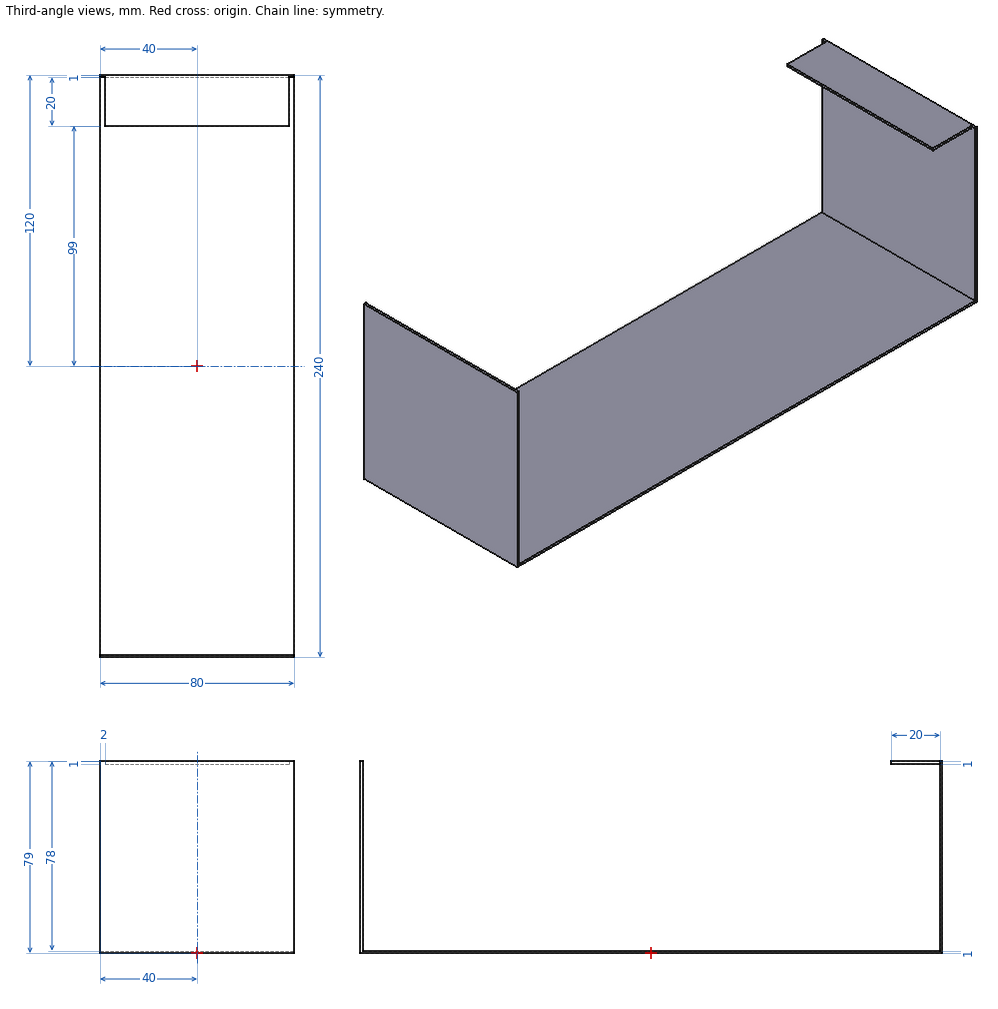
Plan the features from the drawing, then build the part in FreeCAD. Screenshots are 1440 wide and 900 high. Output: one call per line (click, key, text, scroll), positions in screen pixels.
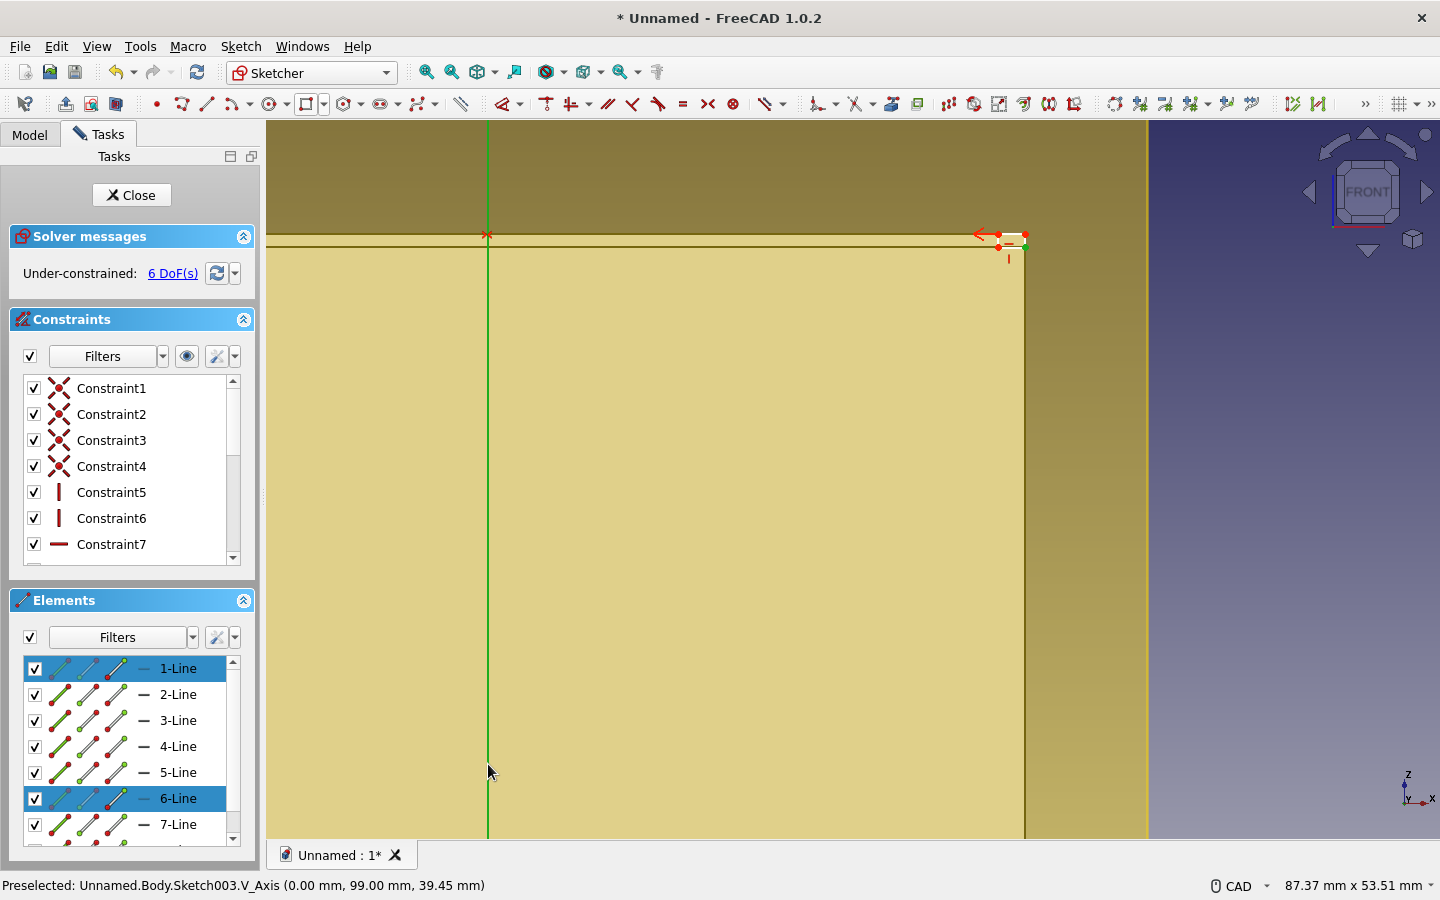
click(708, 104)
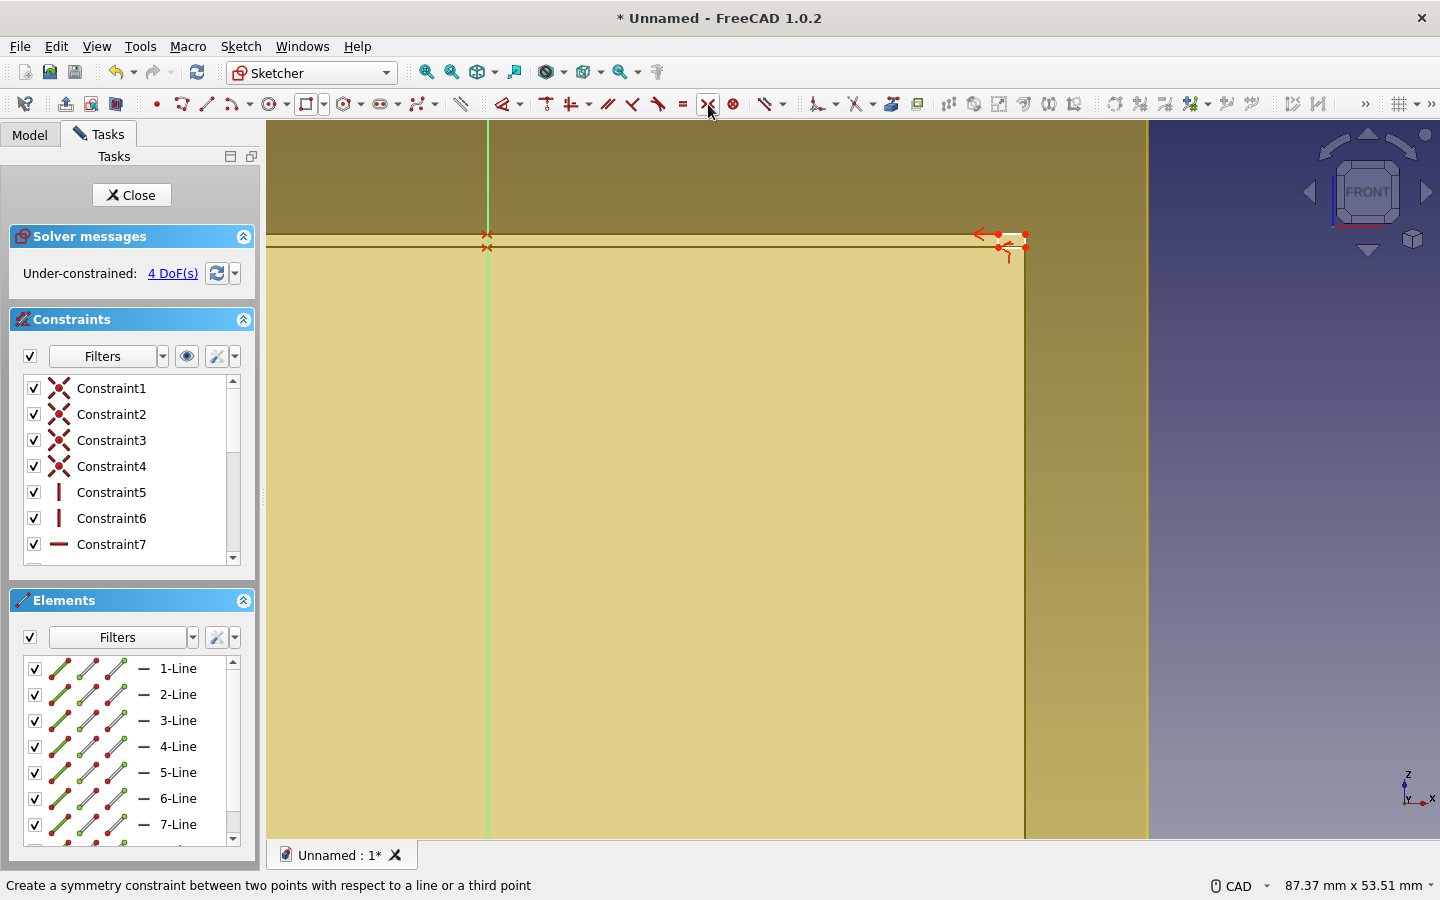
click(502, 104)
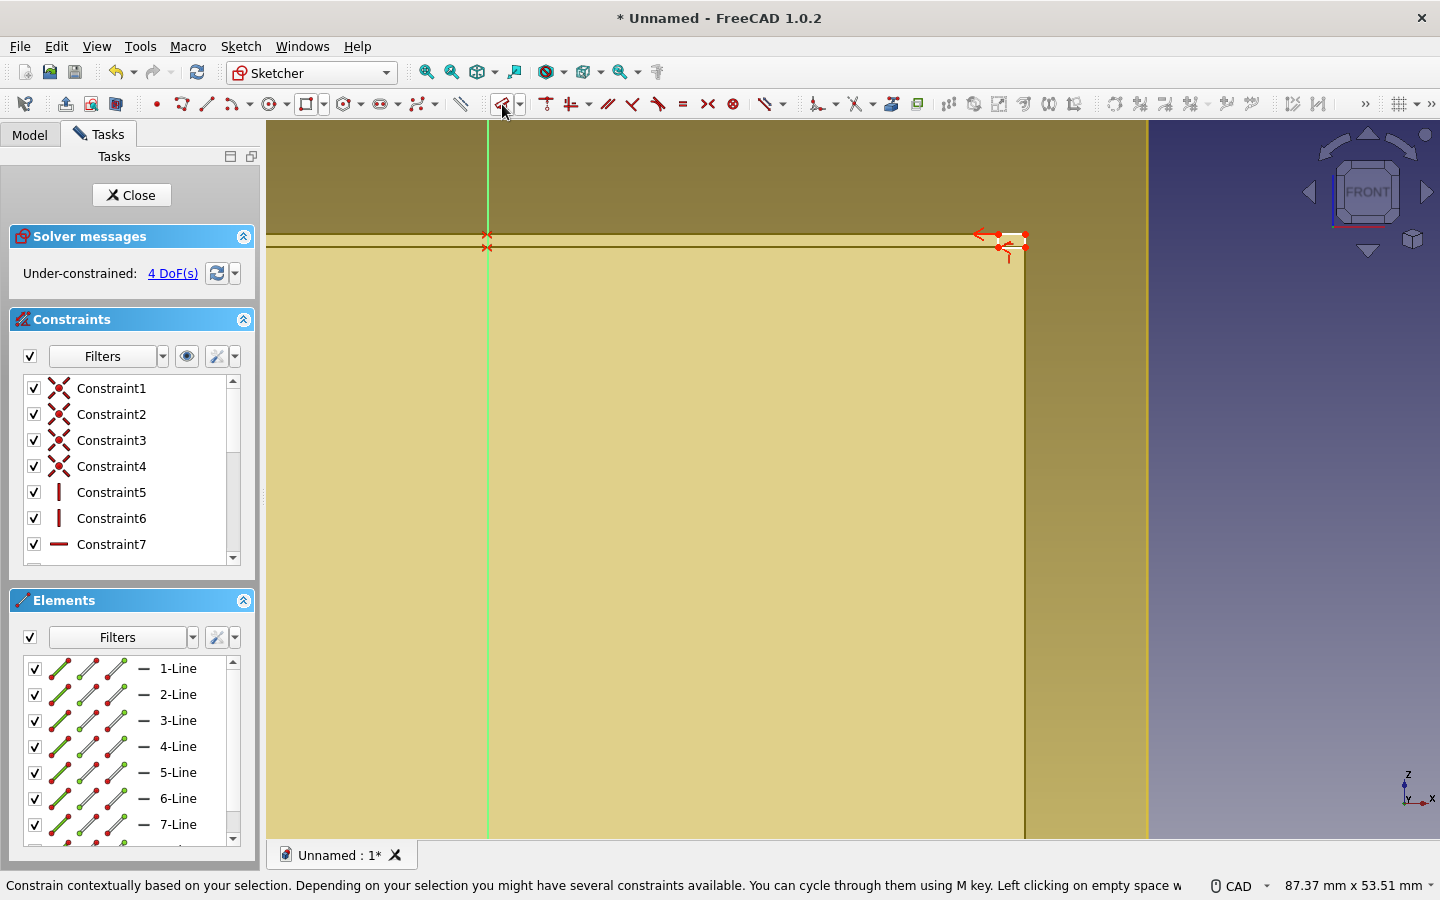
scroll(1027, 247, down, 4)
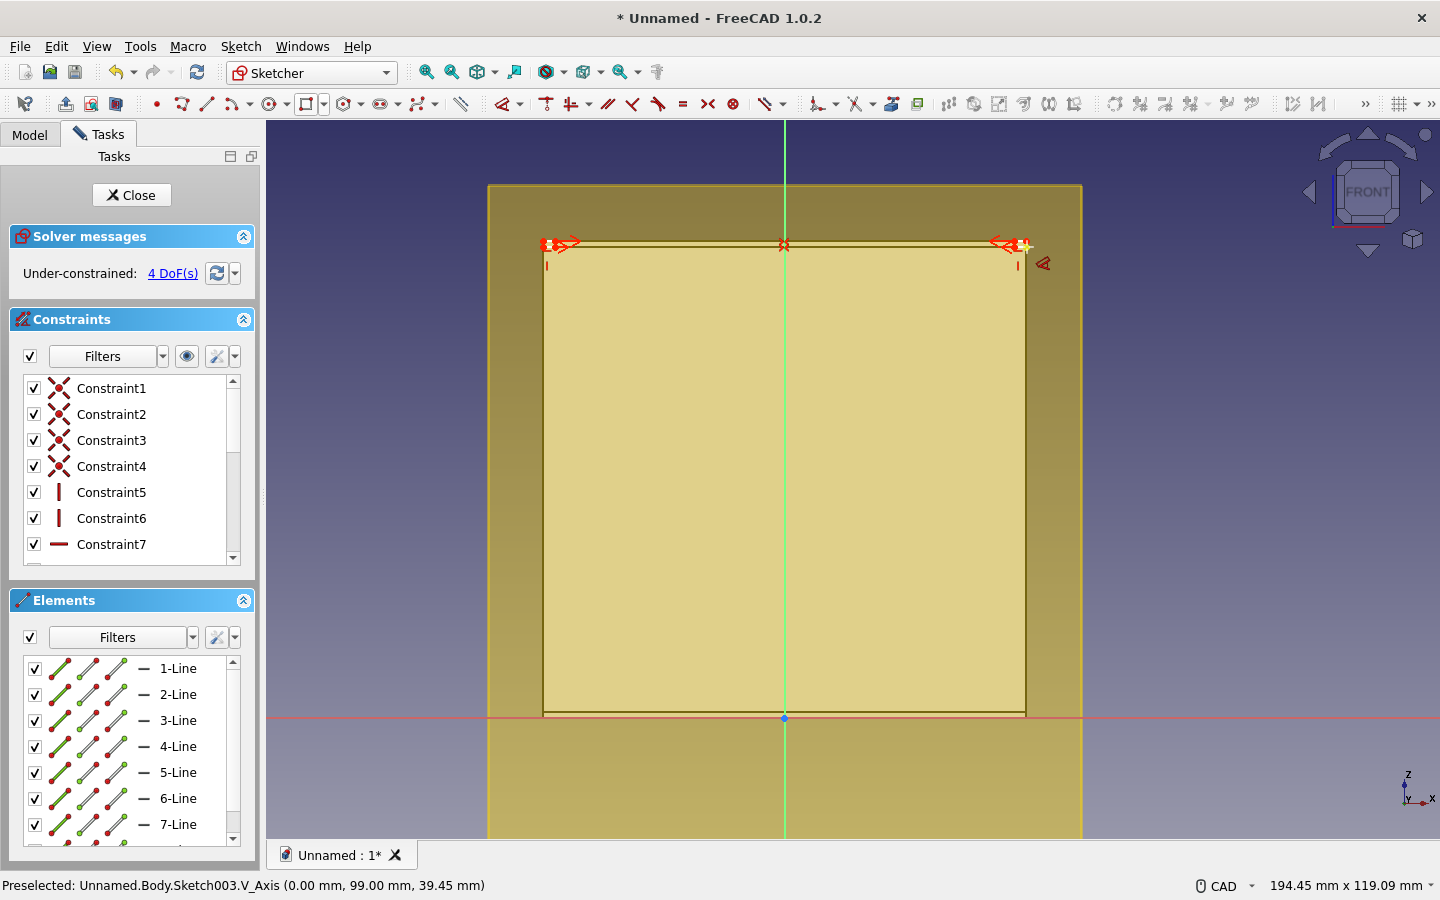
scroll(543, 244, up, 10)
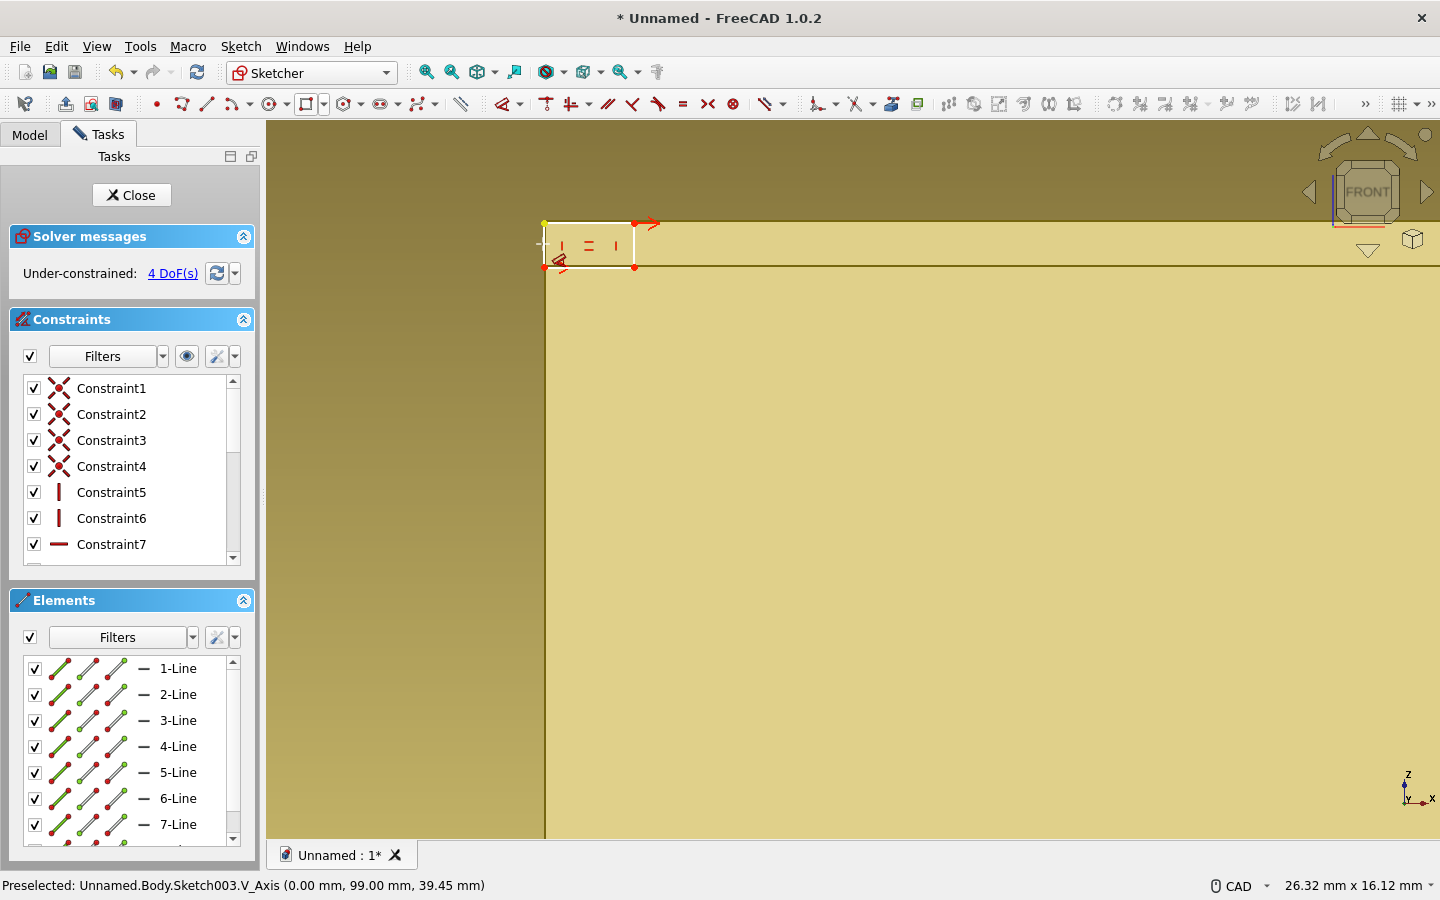
click(544, 246)
click(510, 246)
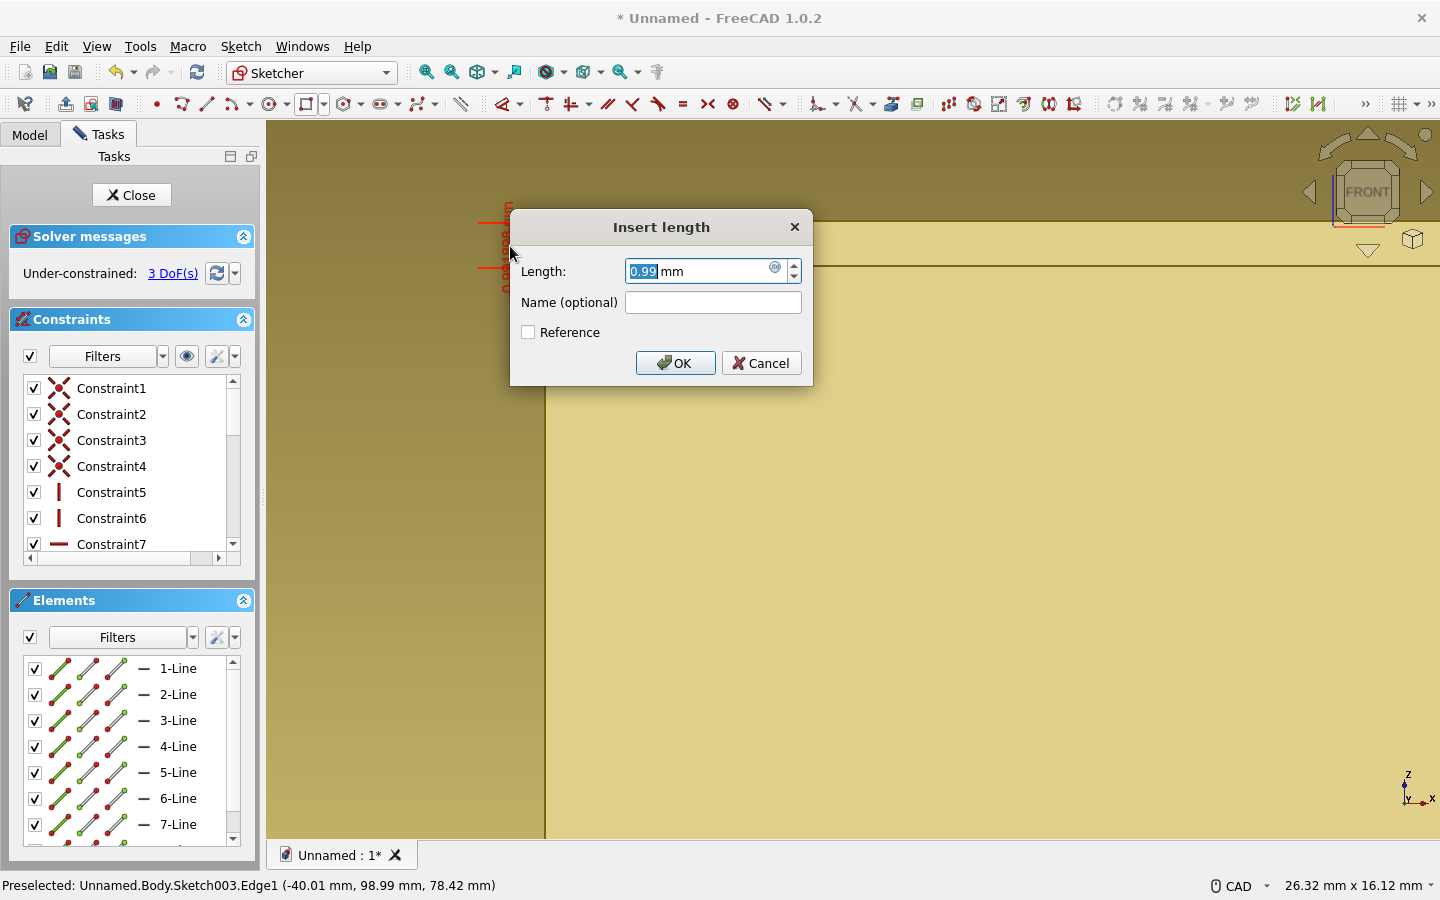
text(1)
key(Return)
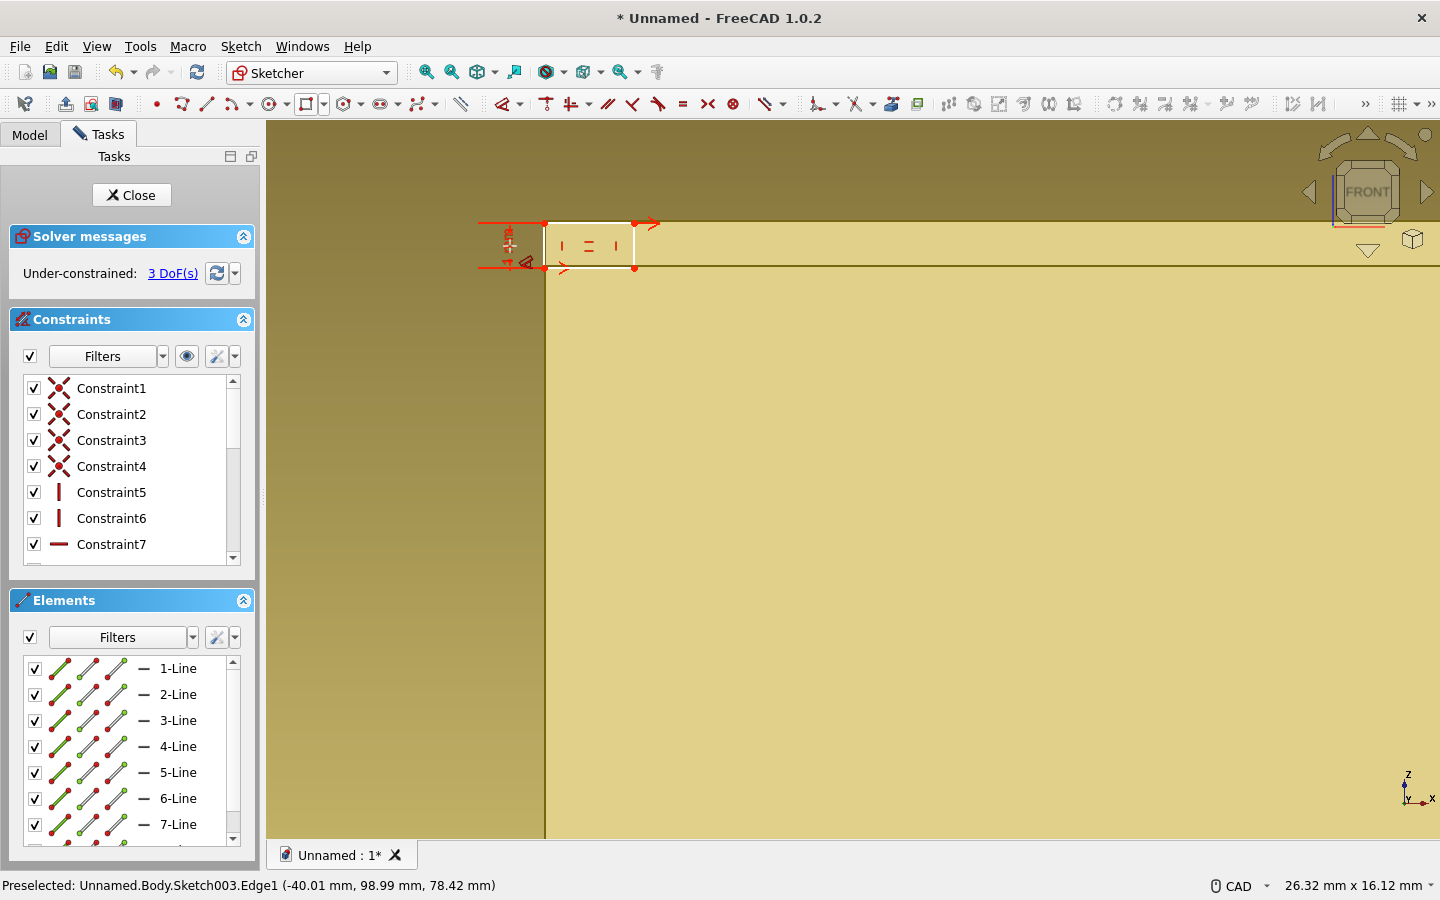
click(571, 268)
click(589, 302)